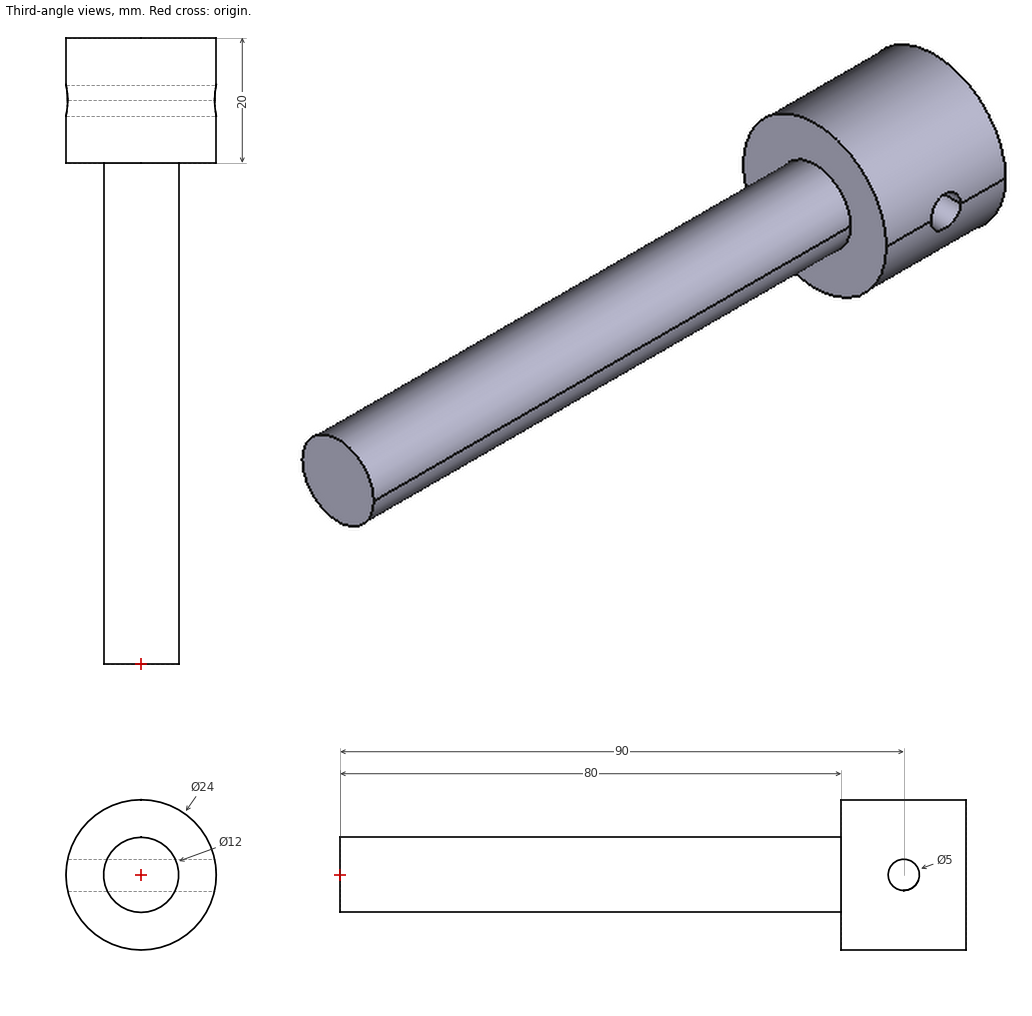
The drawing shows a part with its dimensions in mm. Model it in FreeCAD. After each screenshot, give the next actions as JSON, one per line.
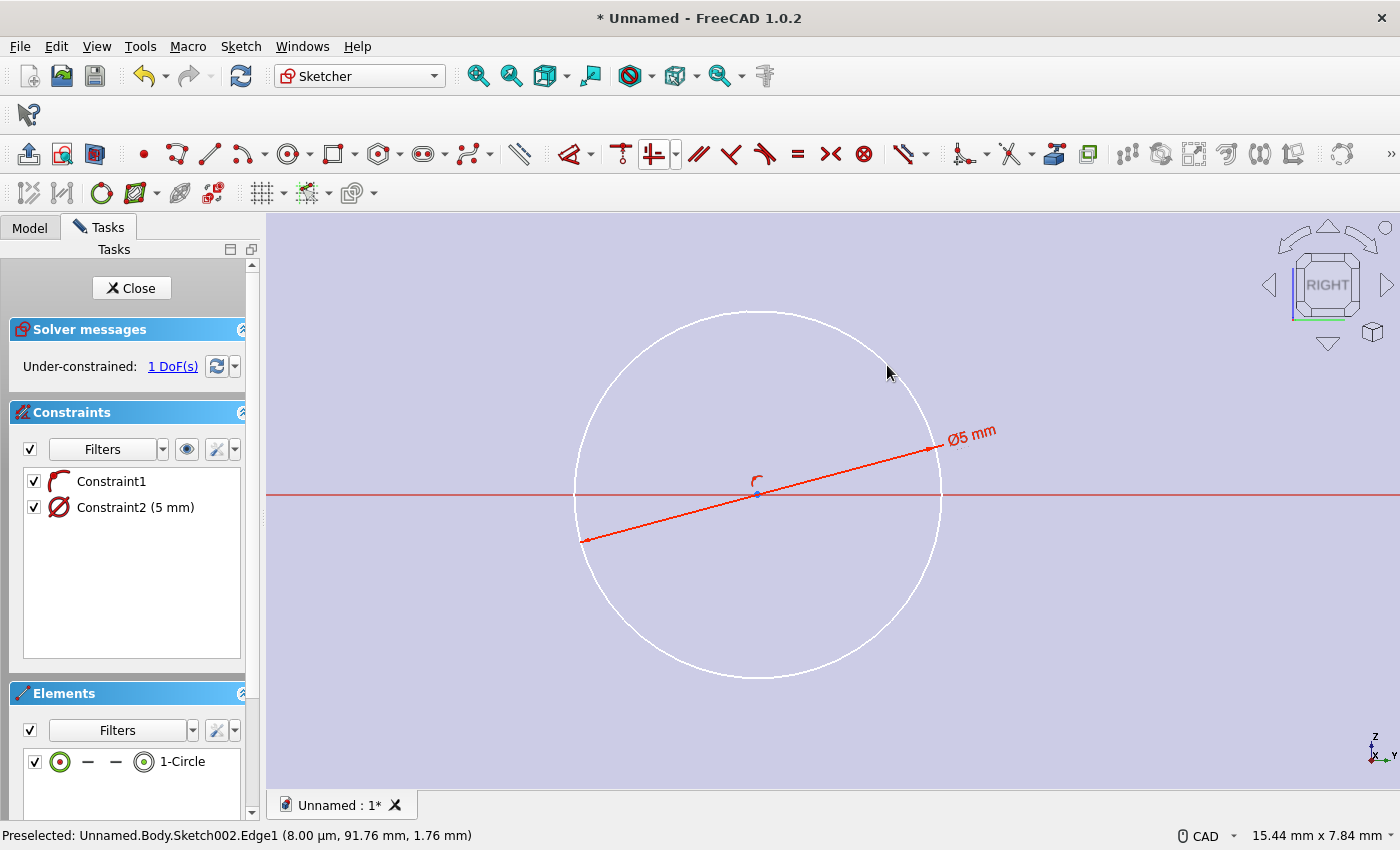
{"action": "left_click", "coordinate": [758, 495]}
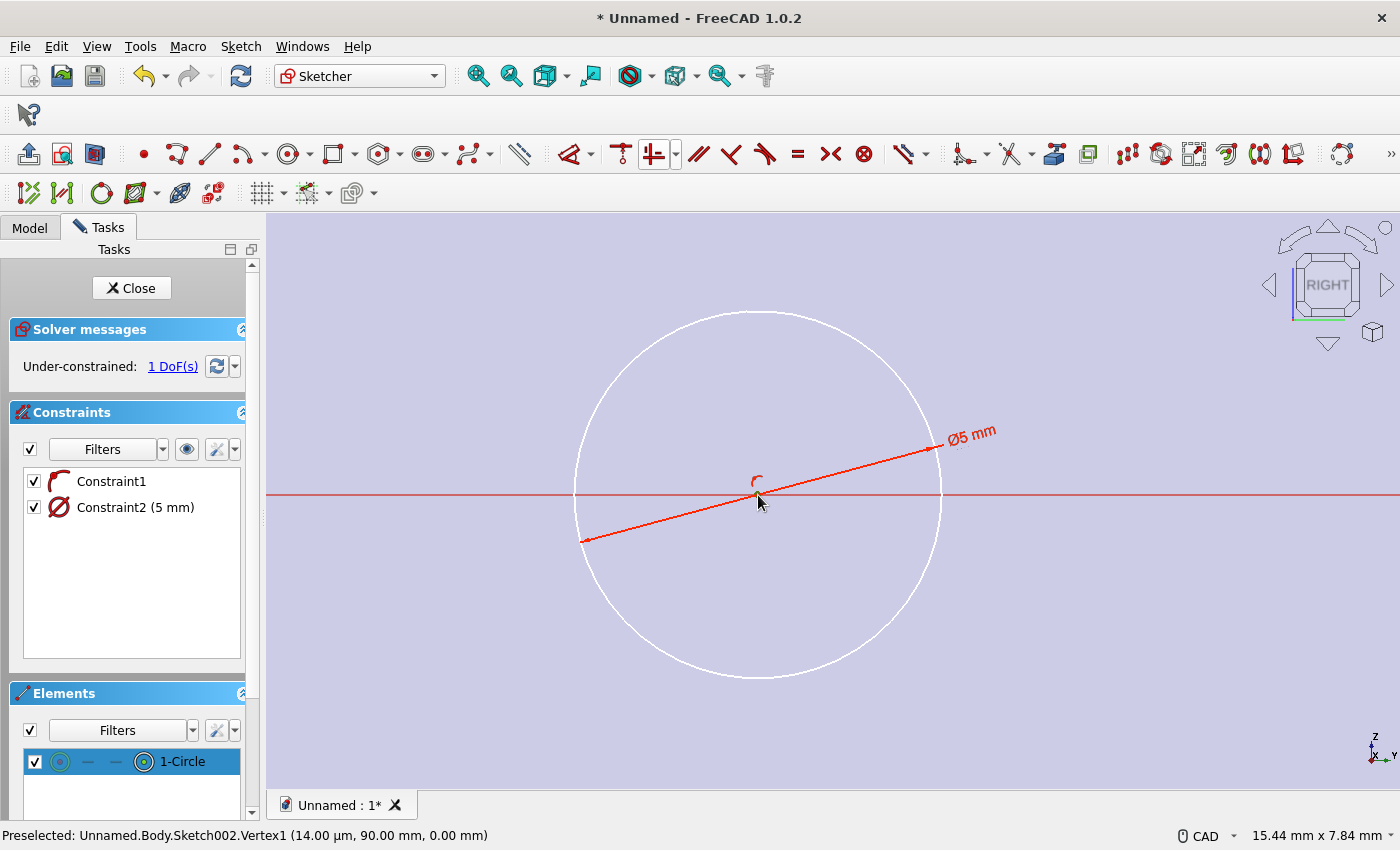
{"action": "key", "text": "l"}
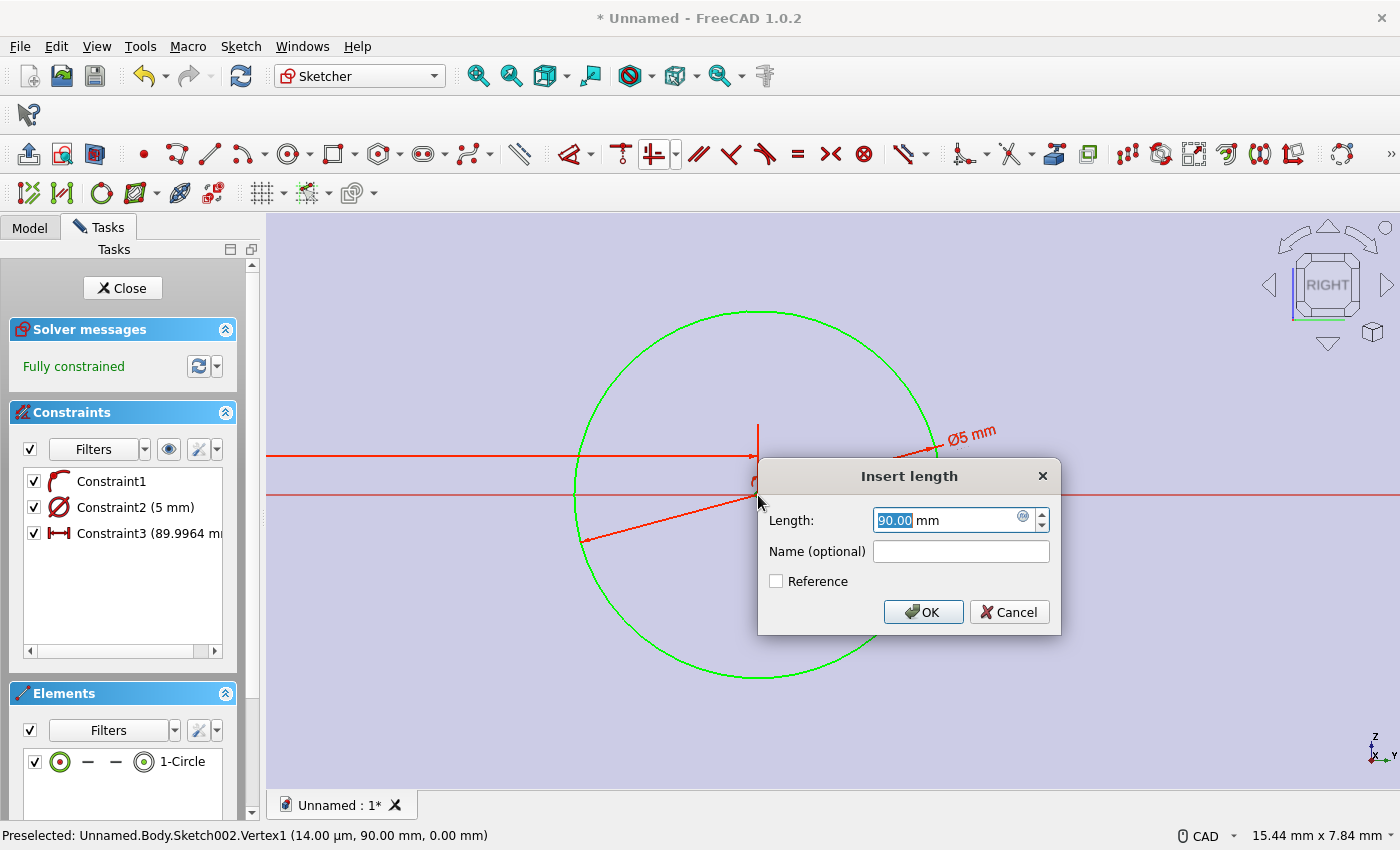
{"action": "type", "text": "90"}
{"action": "key", "text": "Return"}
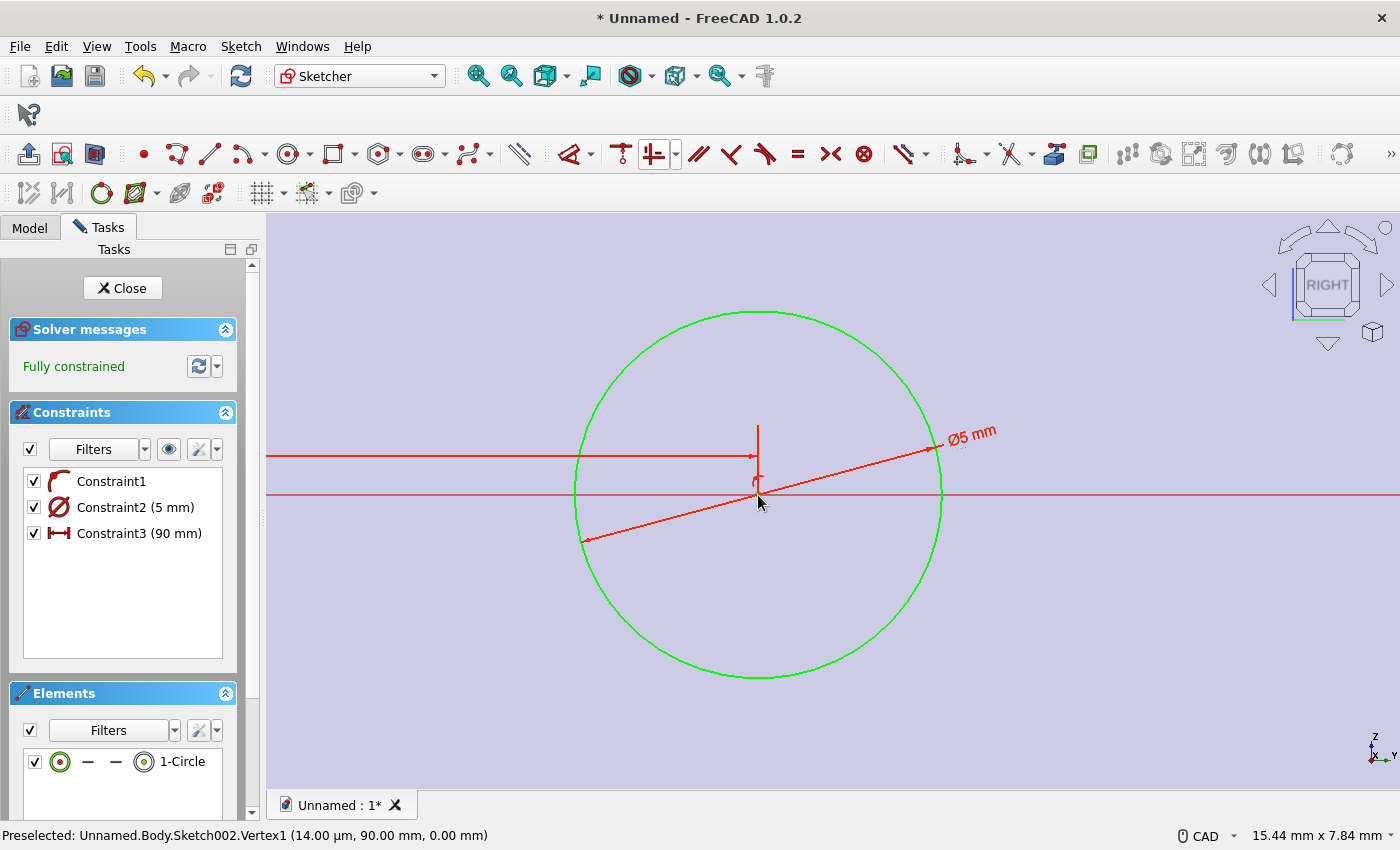
{"action": "left_click", "coordinate": [123, 288]}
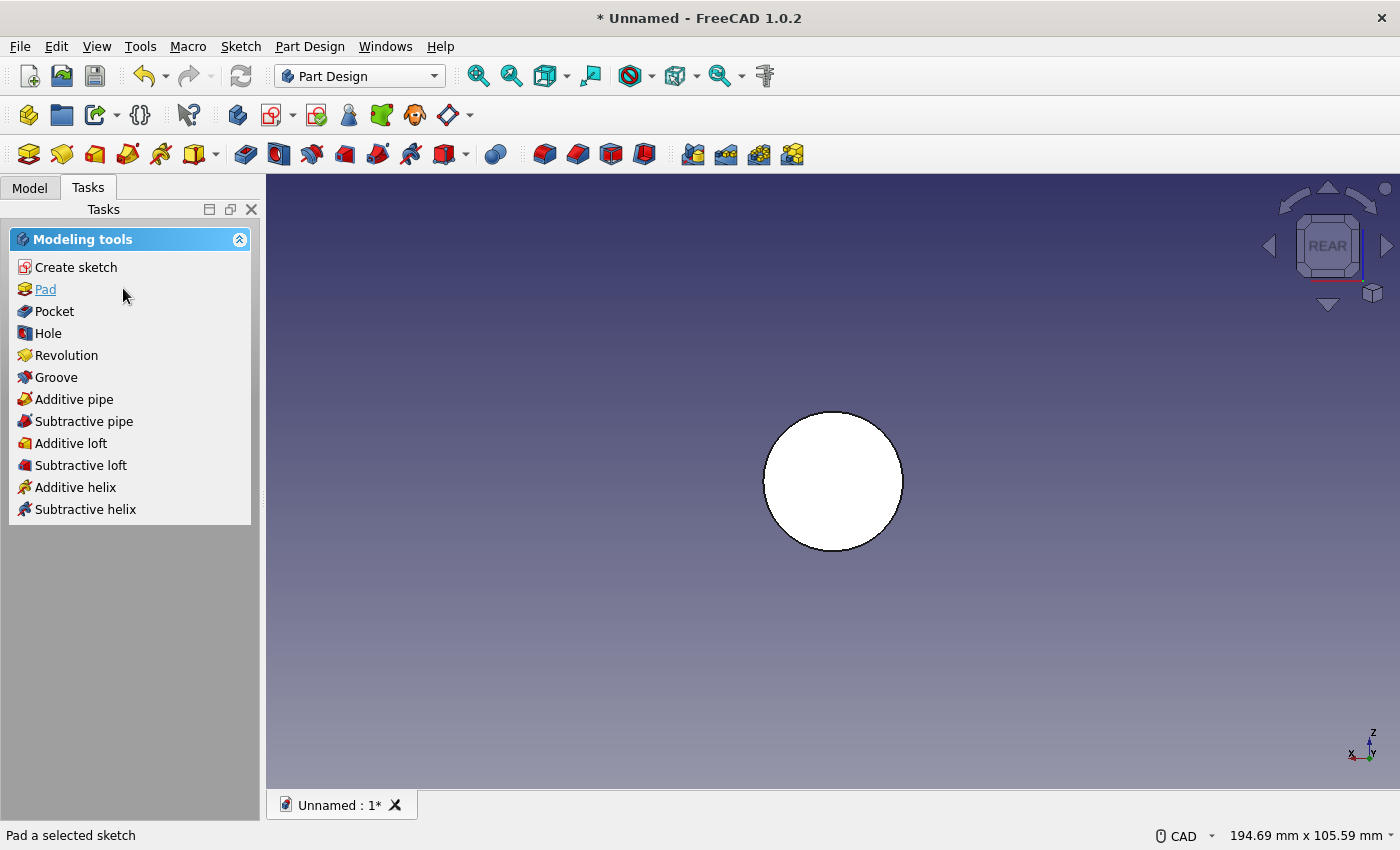
{"action": "left_click", "coordinate": [246, 154]}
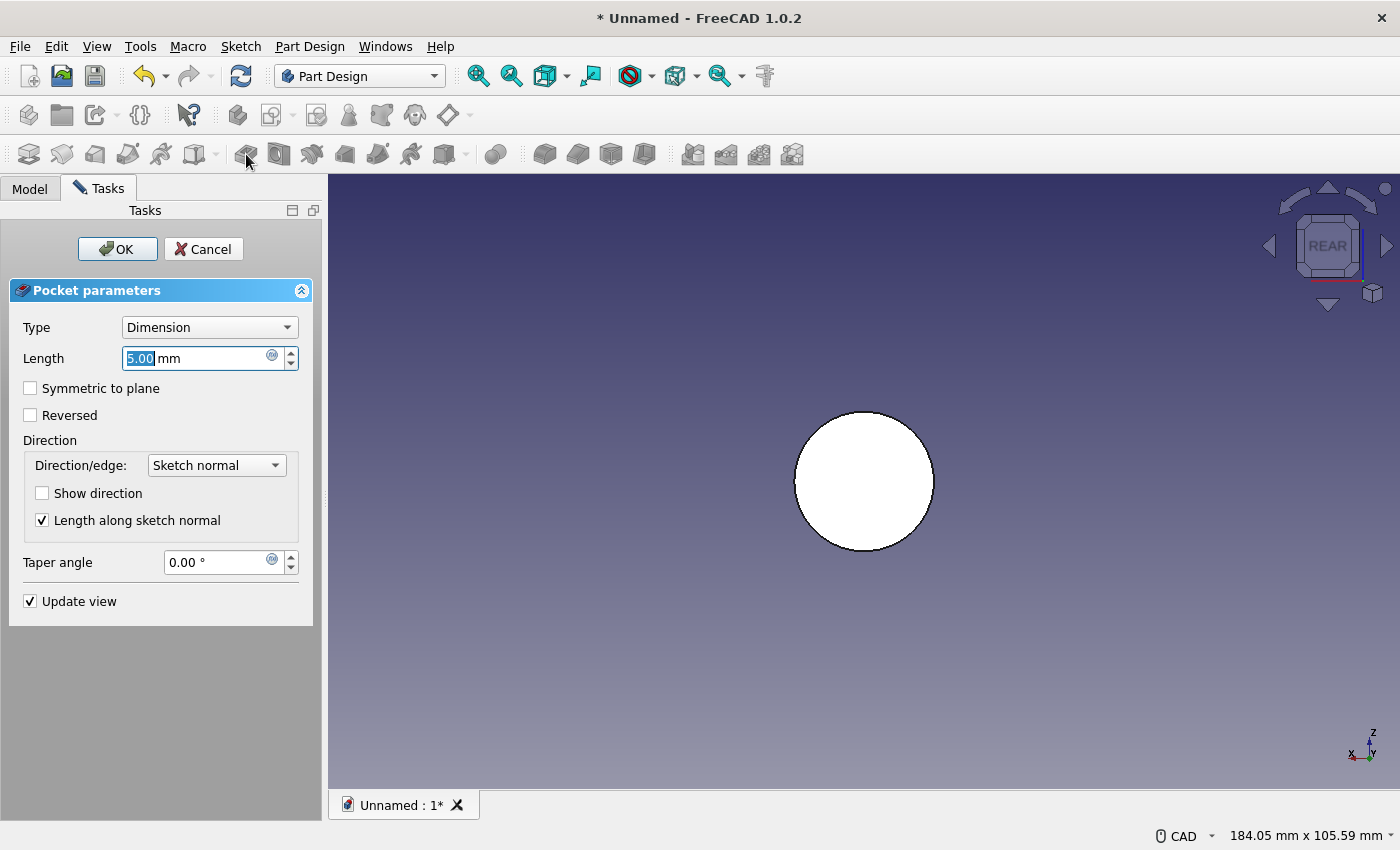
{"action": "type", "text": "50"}
{"action": "key", "text": "Tab"}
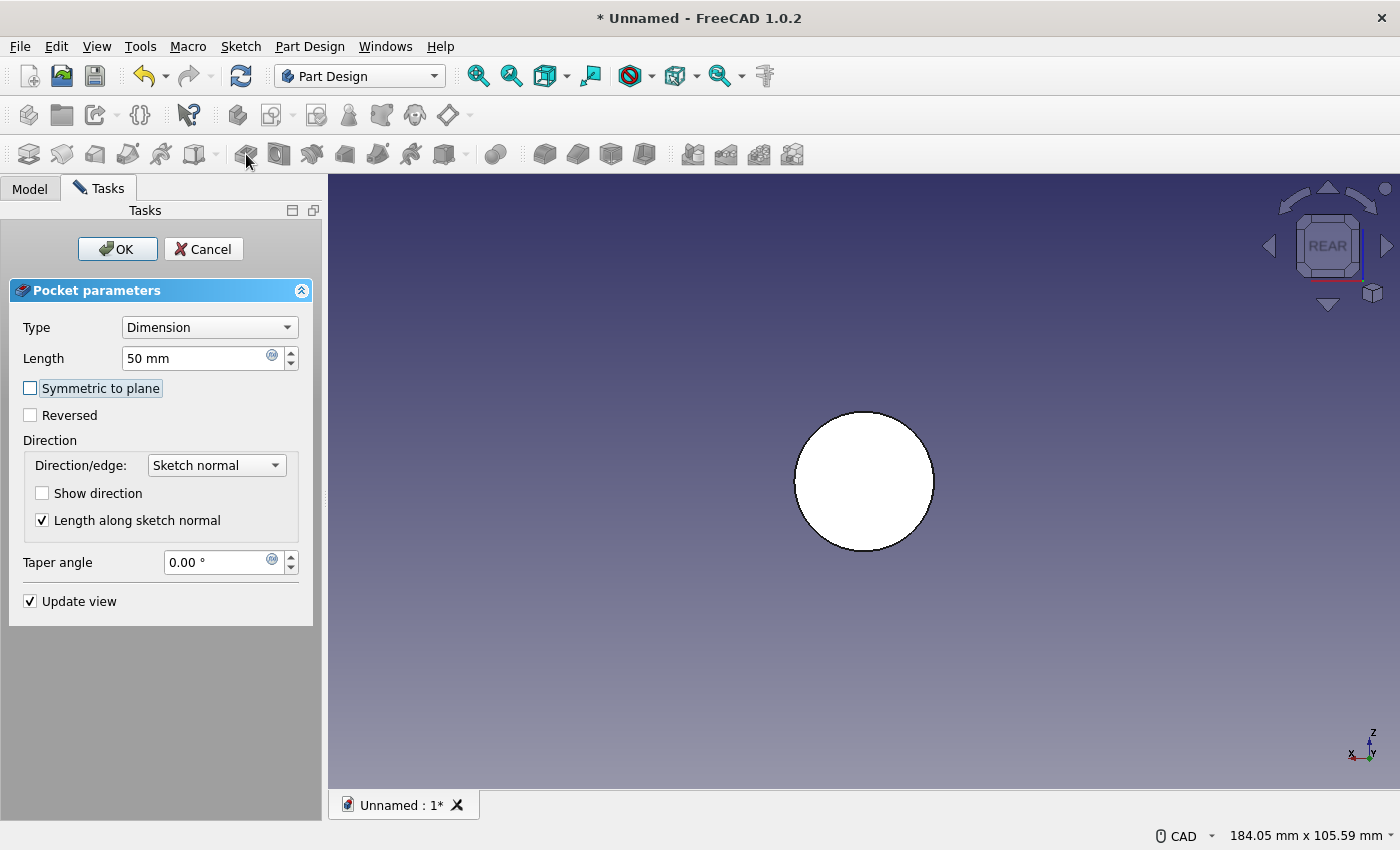
{"action": "left_click", "coordinate": [31, 388]}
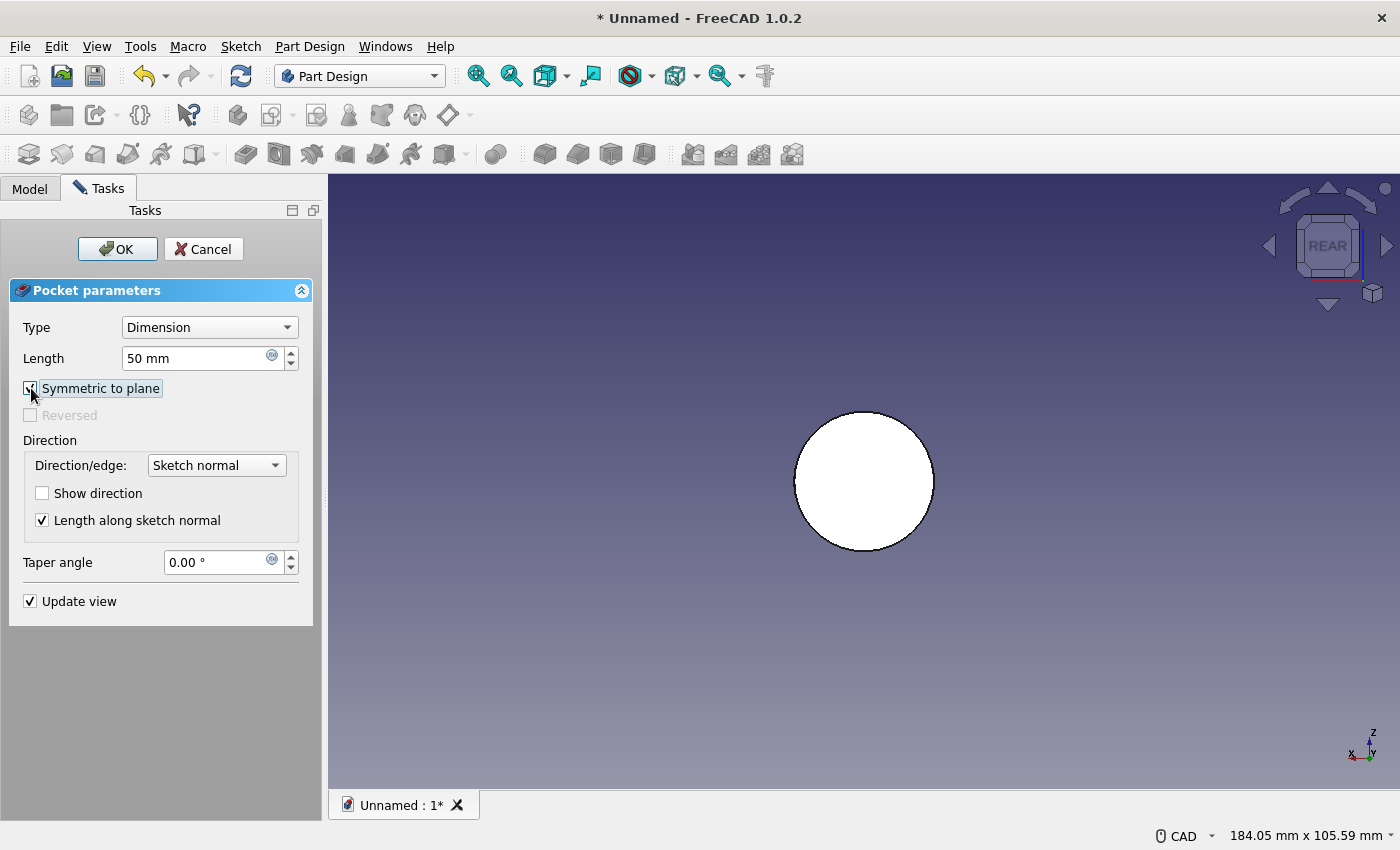
{"action": "left_click", "coordinate": [118, 249]}